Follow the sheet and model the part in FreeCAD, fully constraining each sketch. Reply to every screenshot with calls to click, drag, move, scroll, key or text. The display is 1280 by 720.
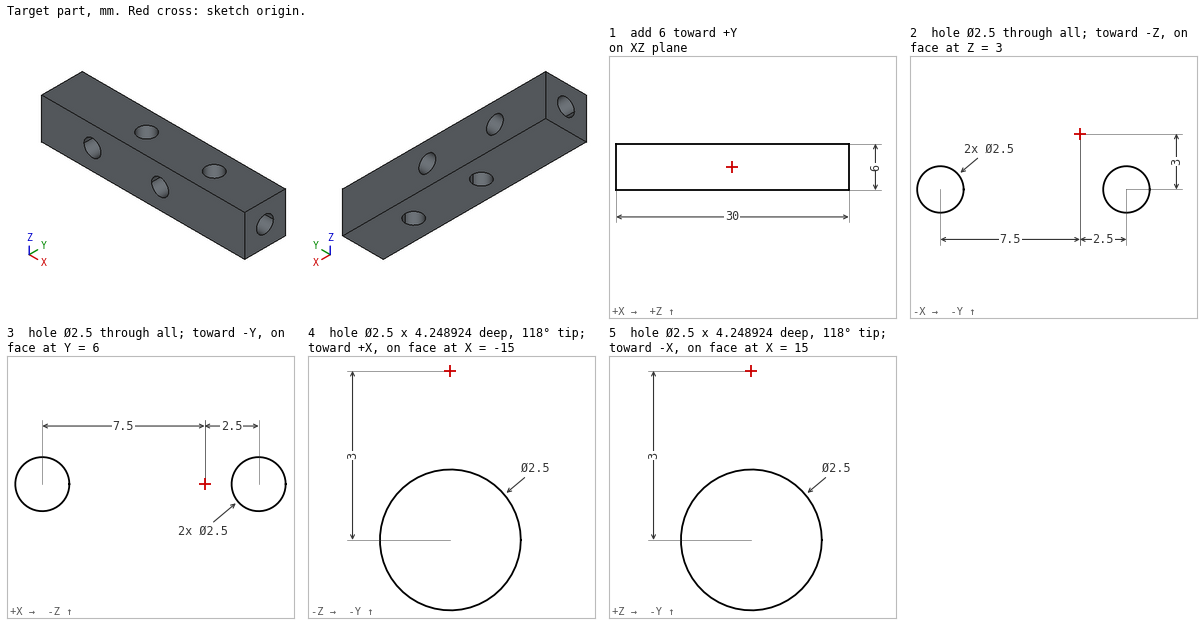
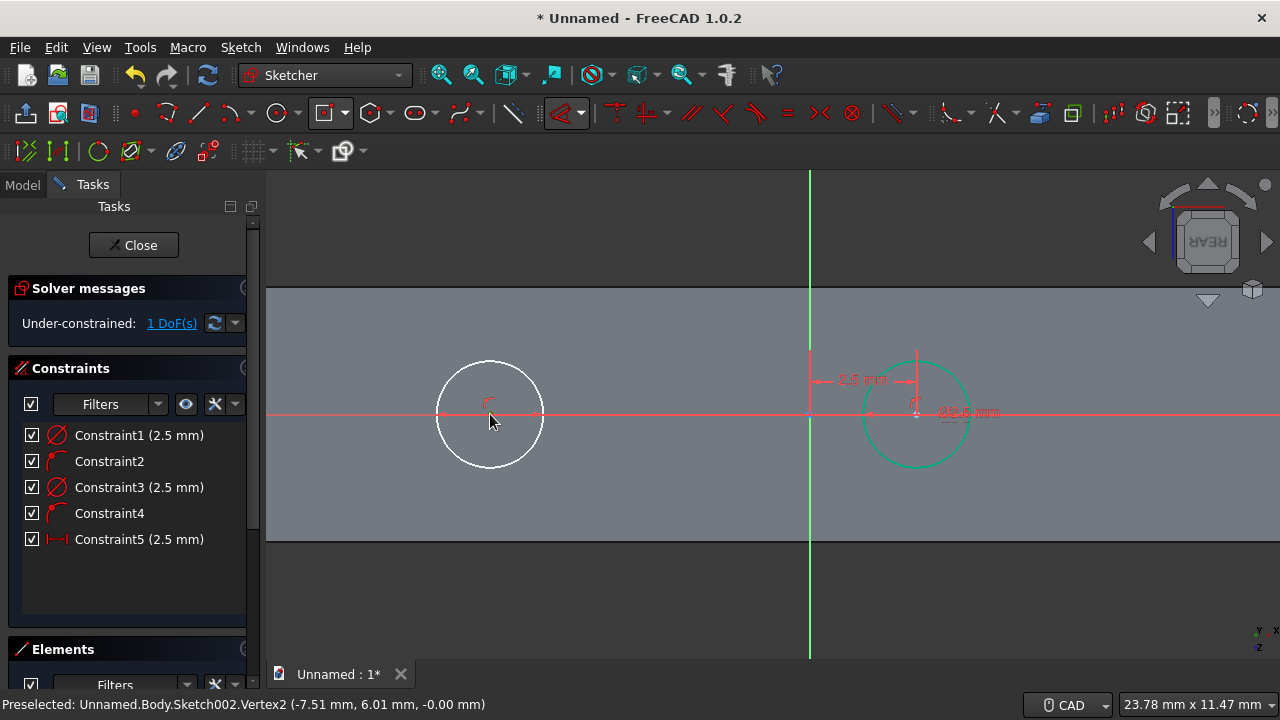
key(l)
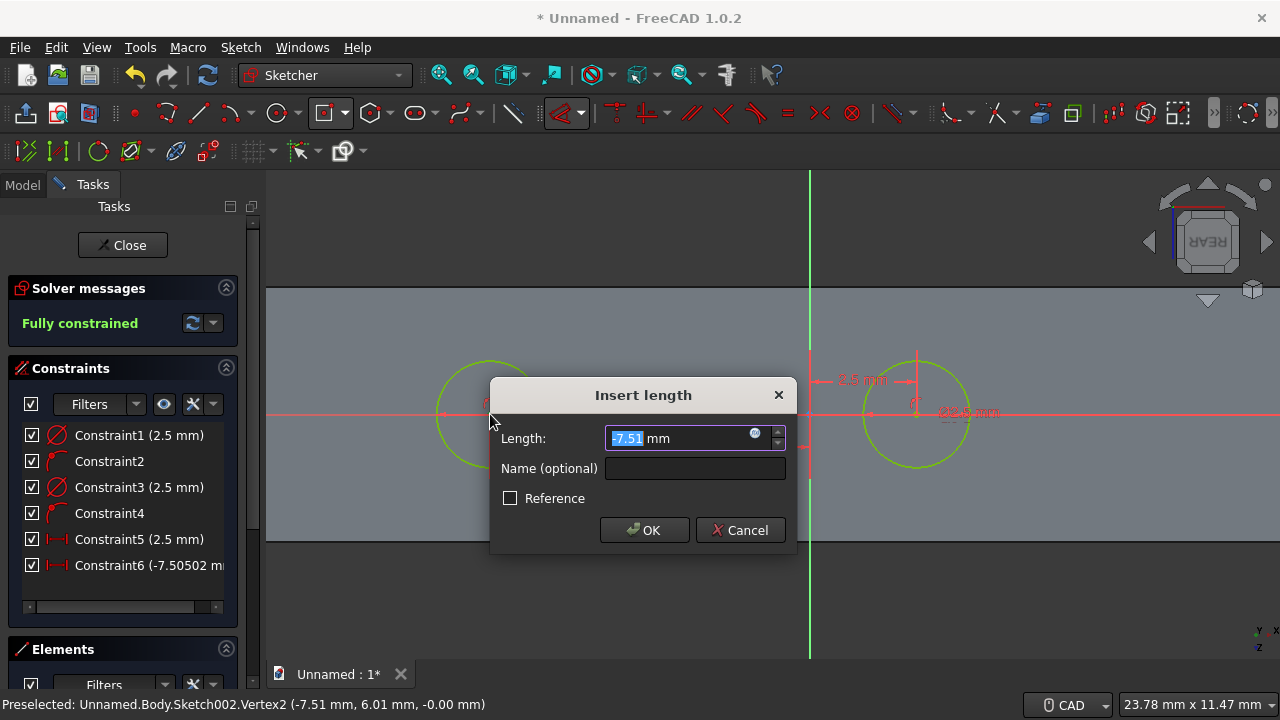
text(-7.5)
key(Return)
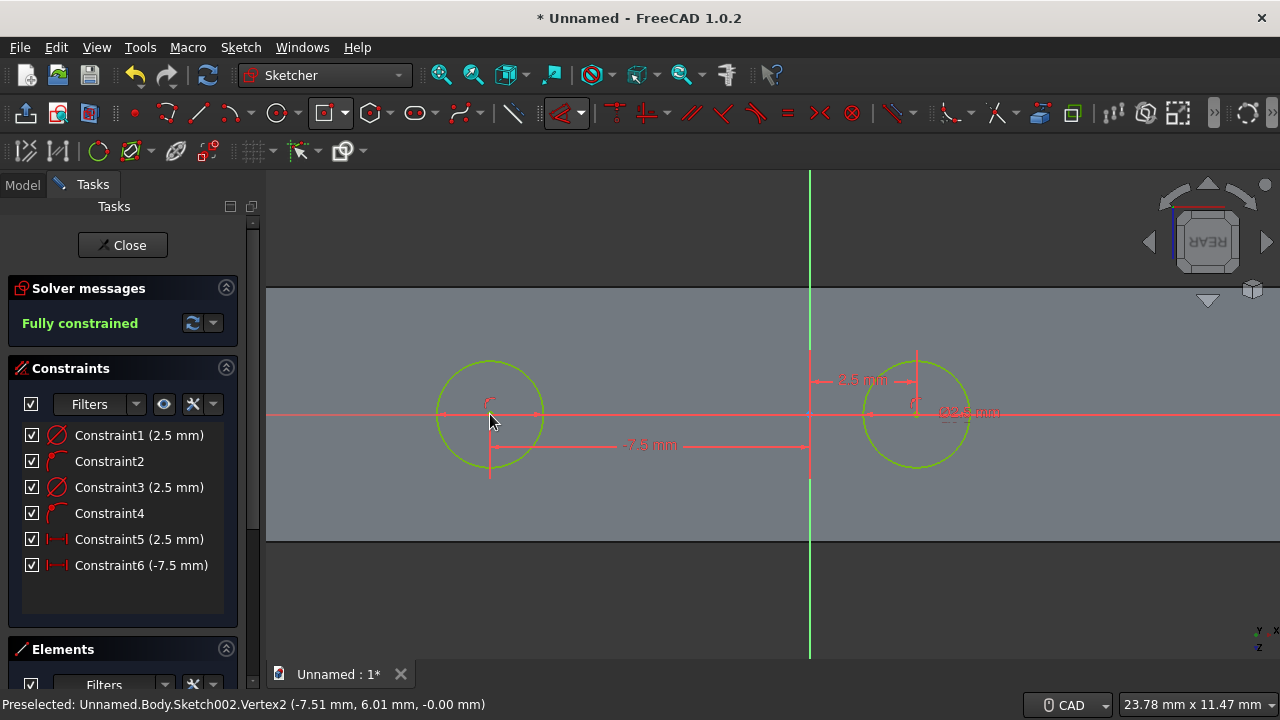
click(123, 245)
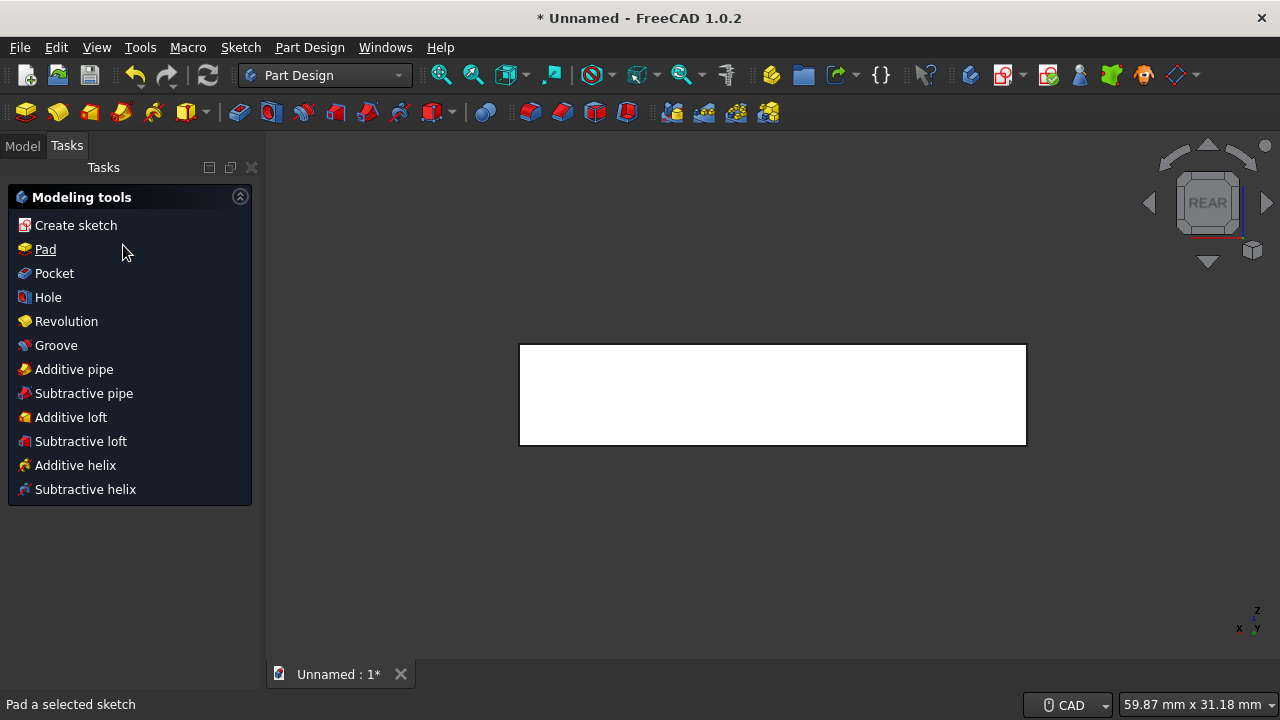
click(272, 112)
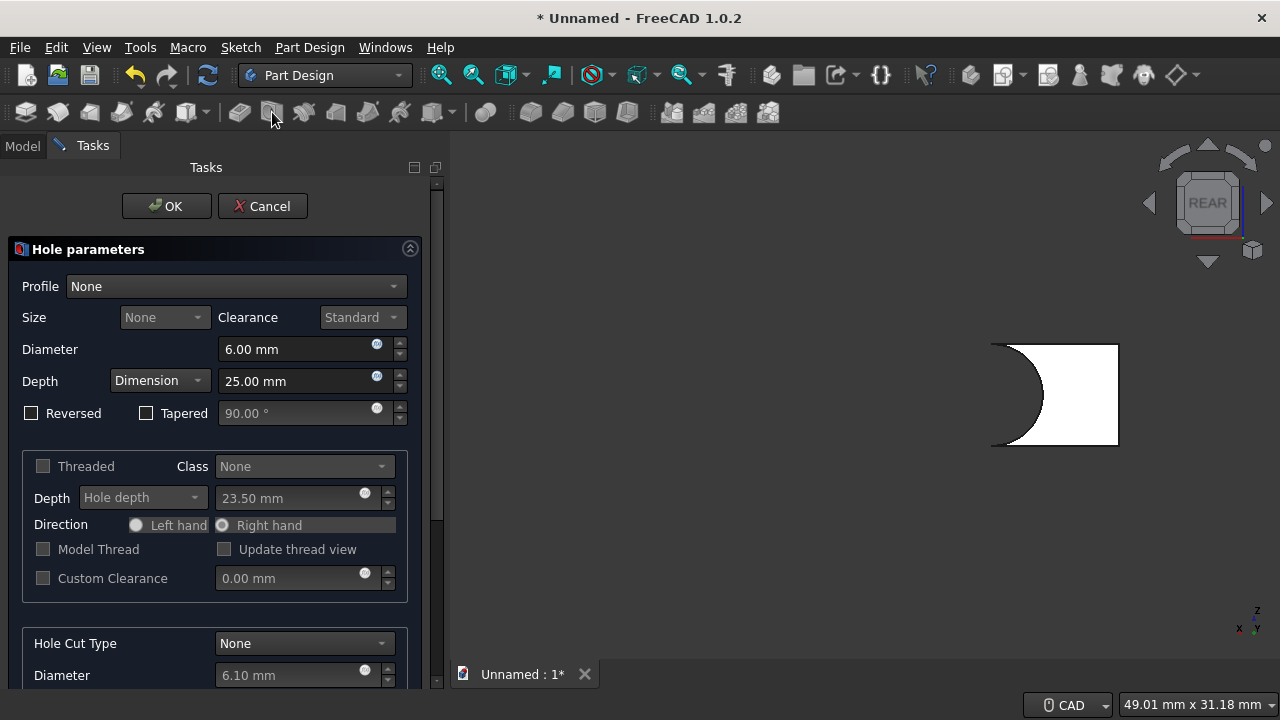
triple_click(305, 349)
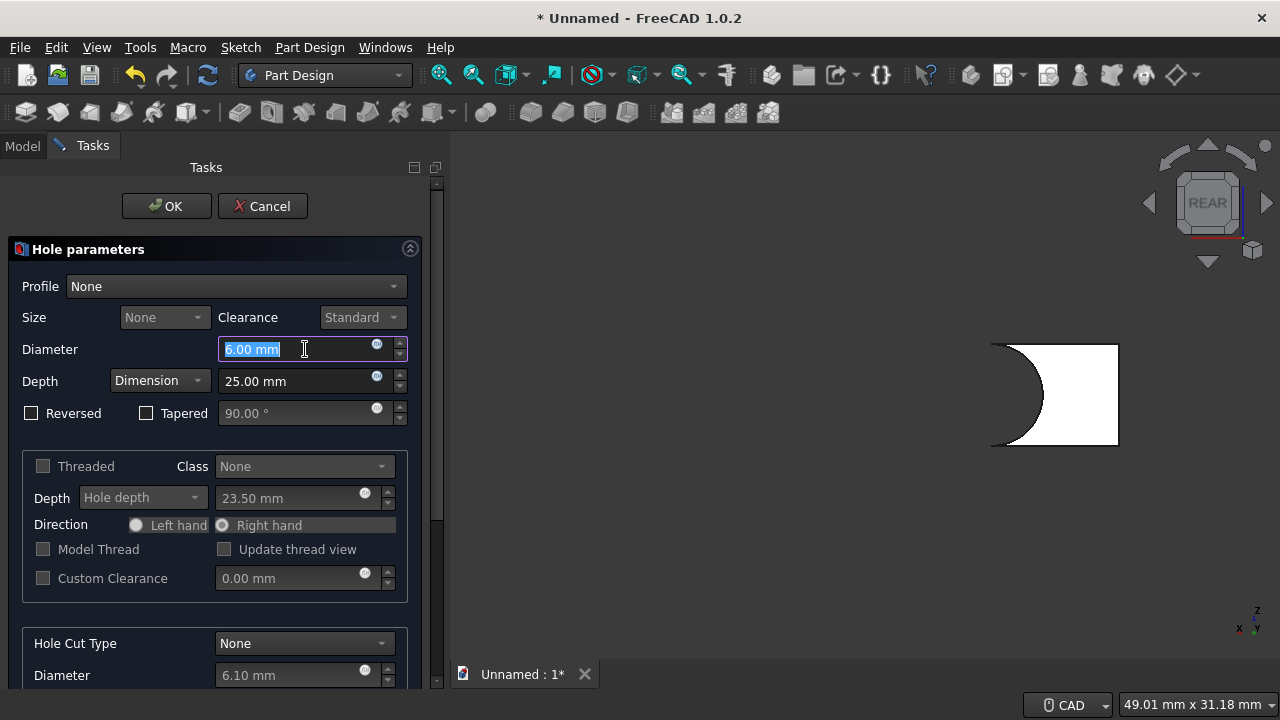
text(2.5)
key(Tab)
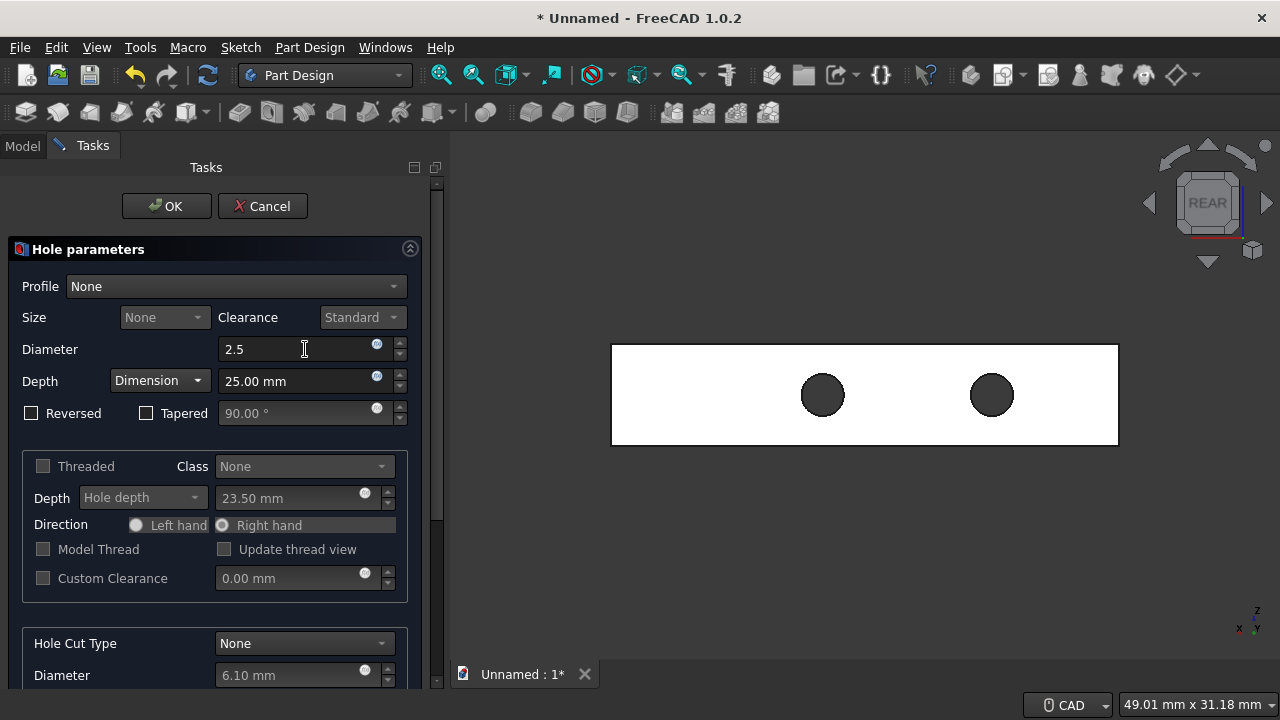
click(161, 380)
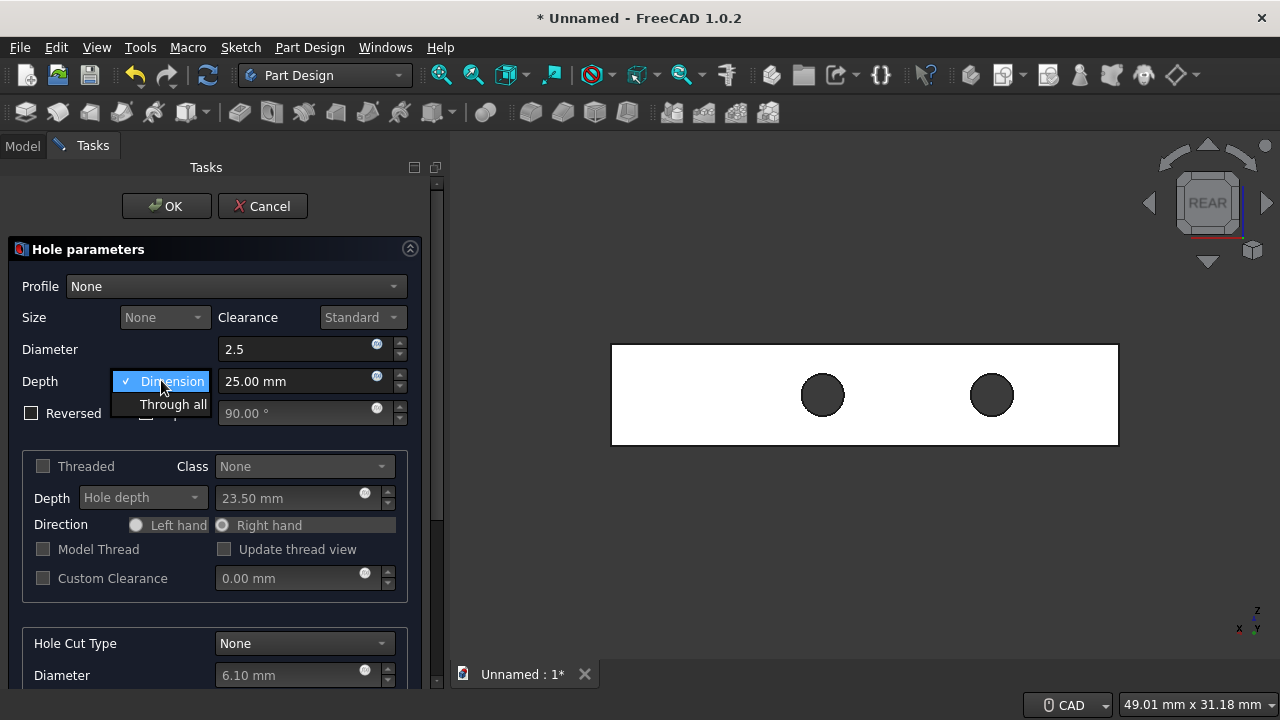
click(160, 404)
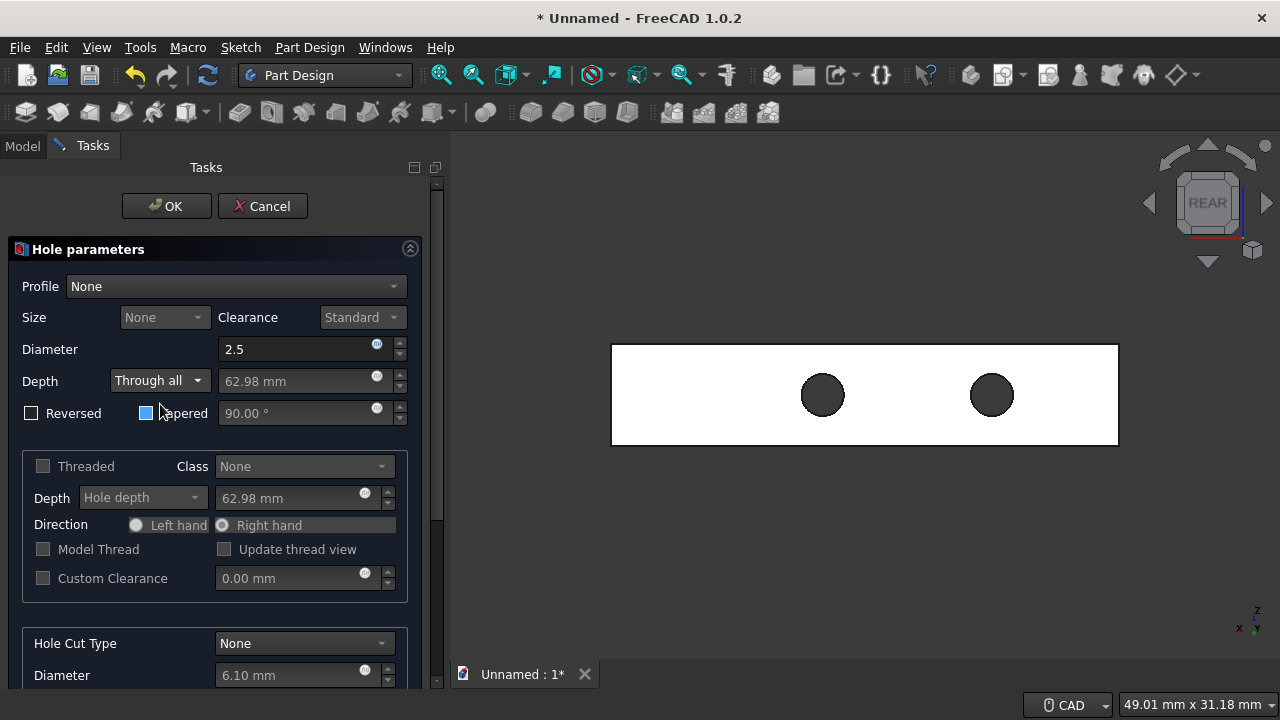
click(167, 206)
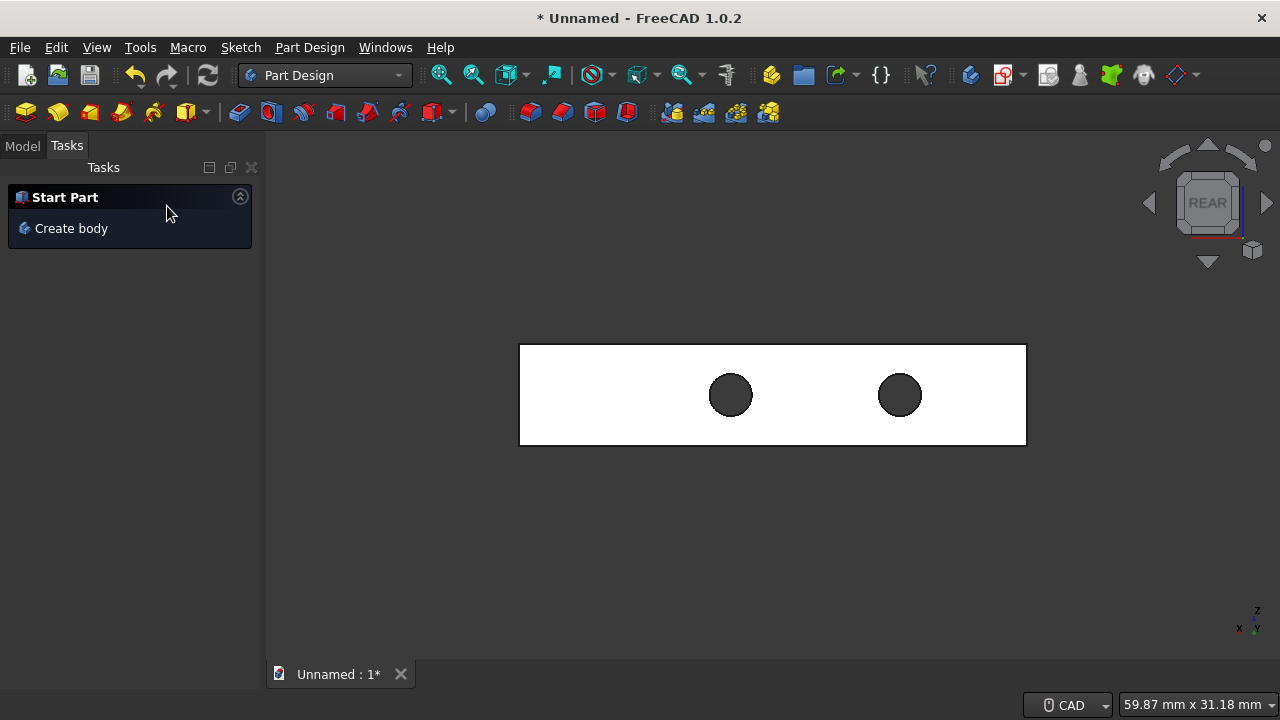
key(6)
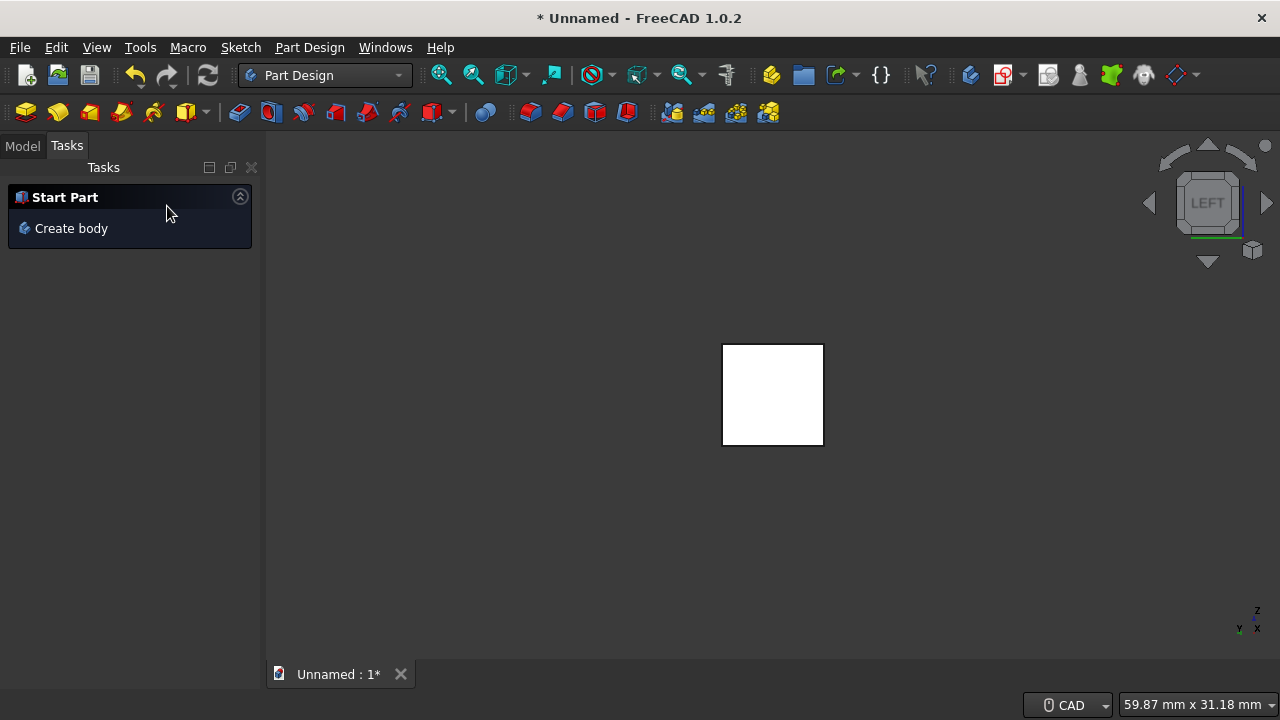
key(v)
key(f)